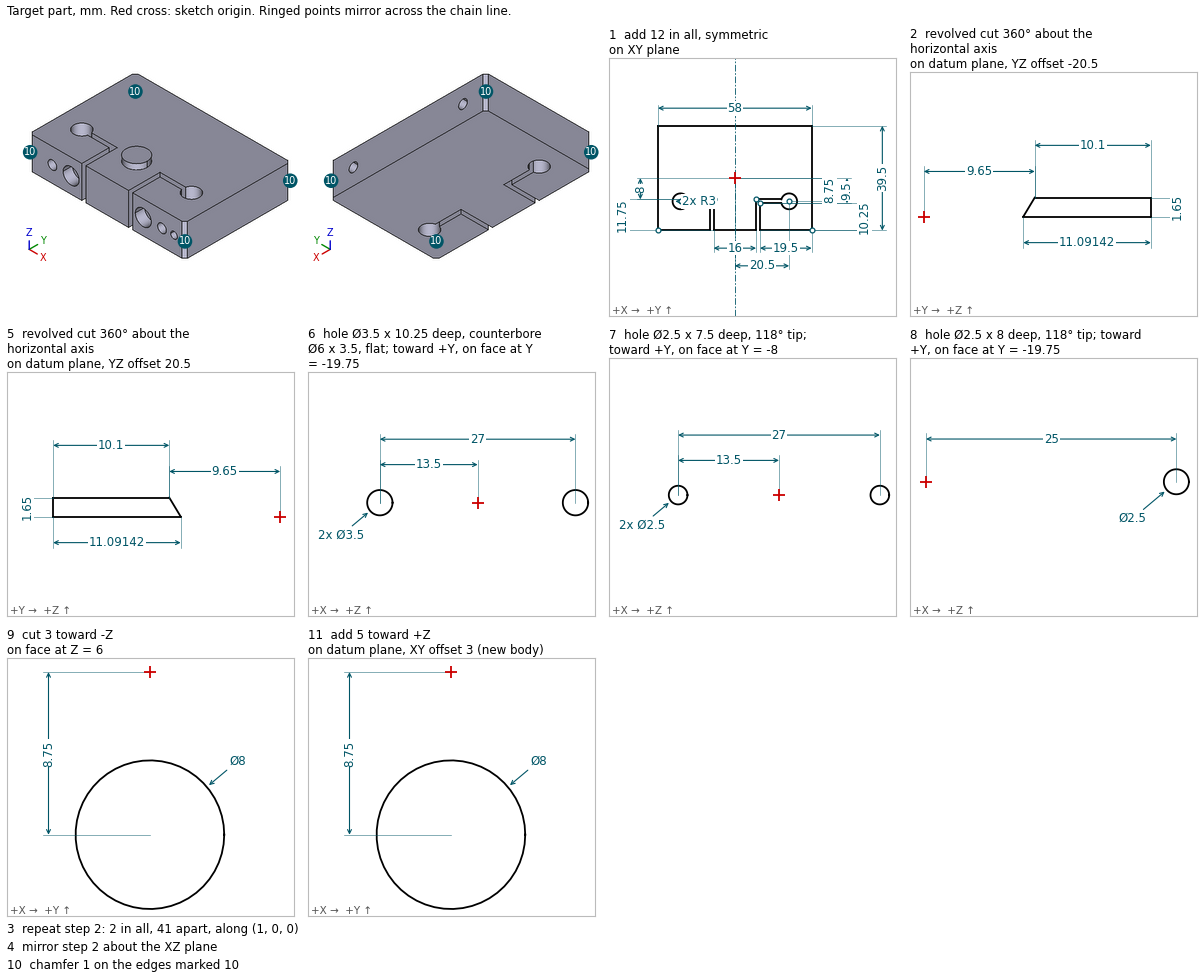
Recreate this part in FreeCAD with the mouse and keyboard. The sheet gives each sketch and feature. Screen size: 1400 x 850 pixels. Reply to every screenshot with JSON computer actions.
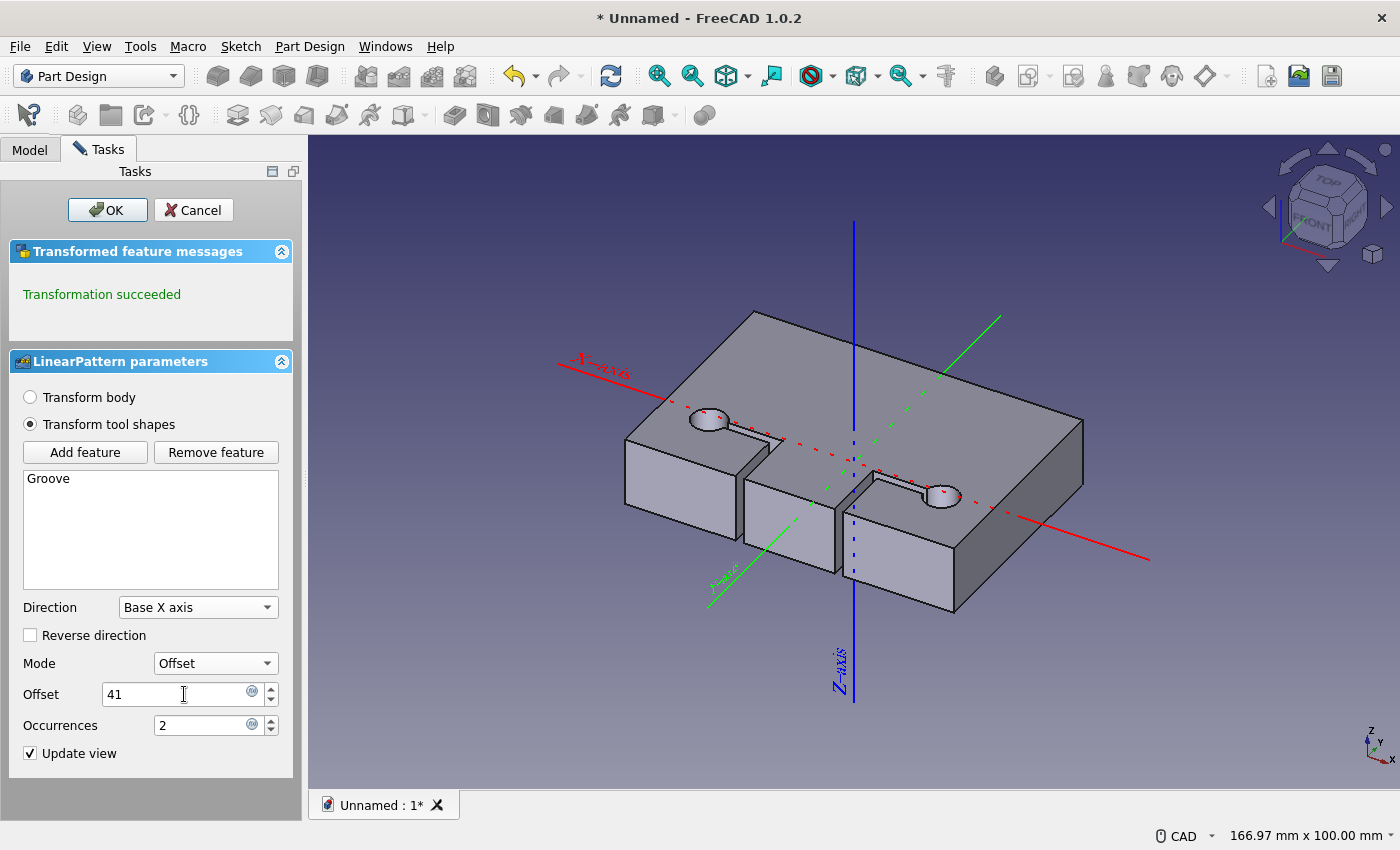
{"action": "triple_click", "coordinate": [210, 726]}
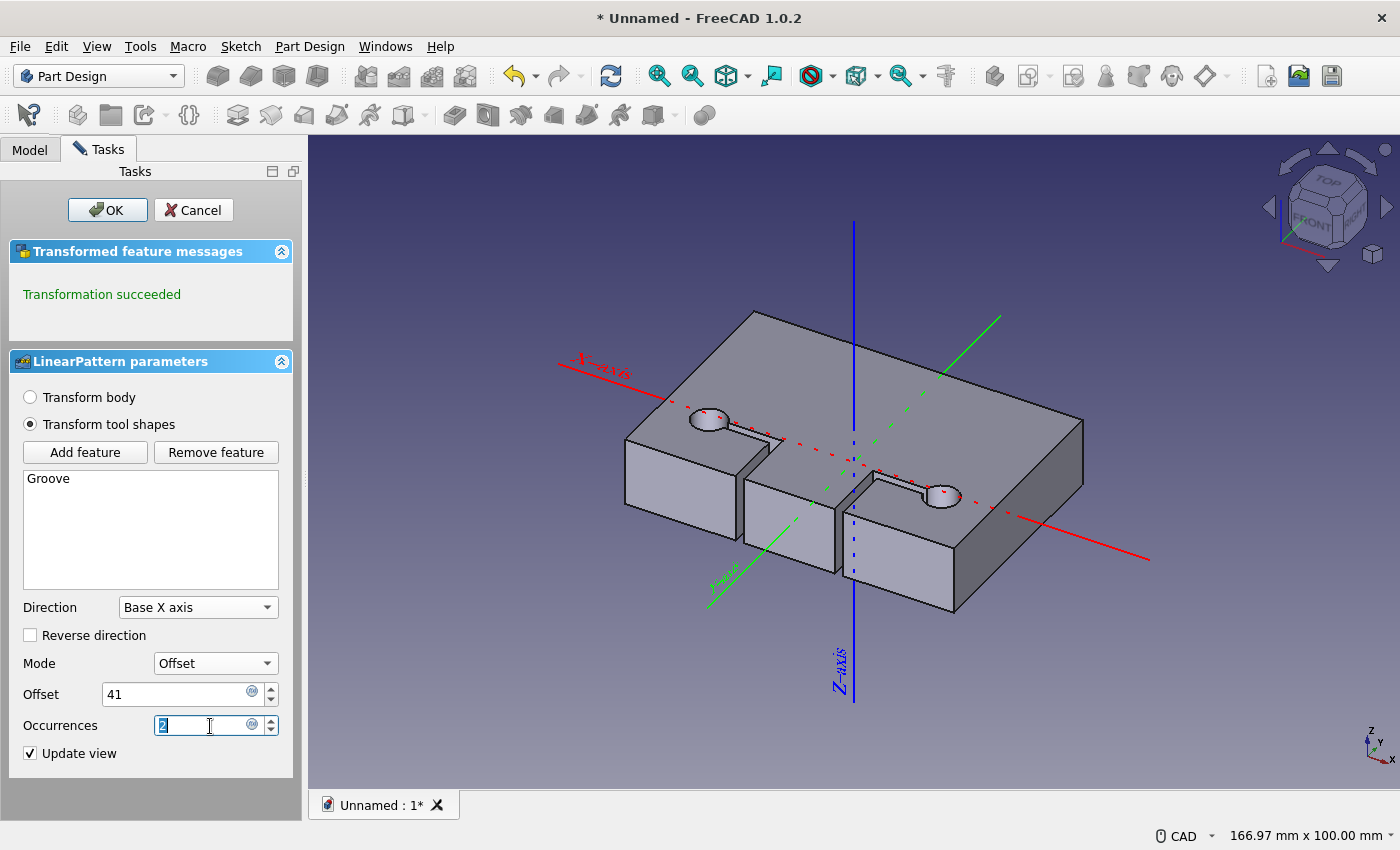
{"action": "type", "text": "2"}
{"action": "key", "text": "Tab"}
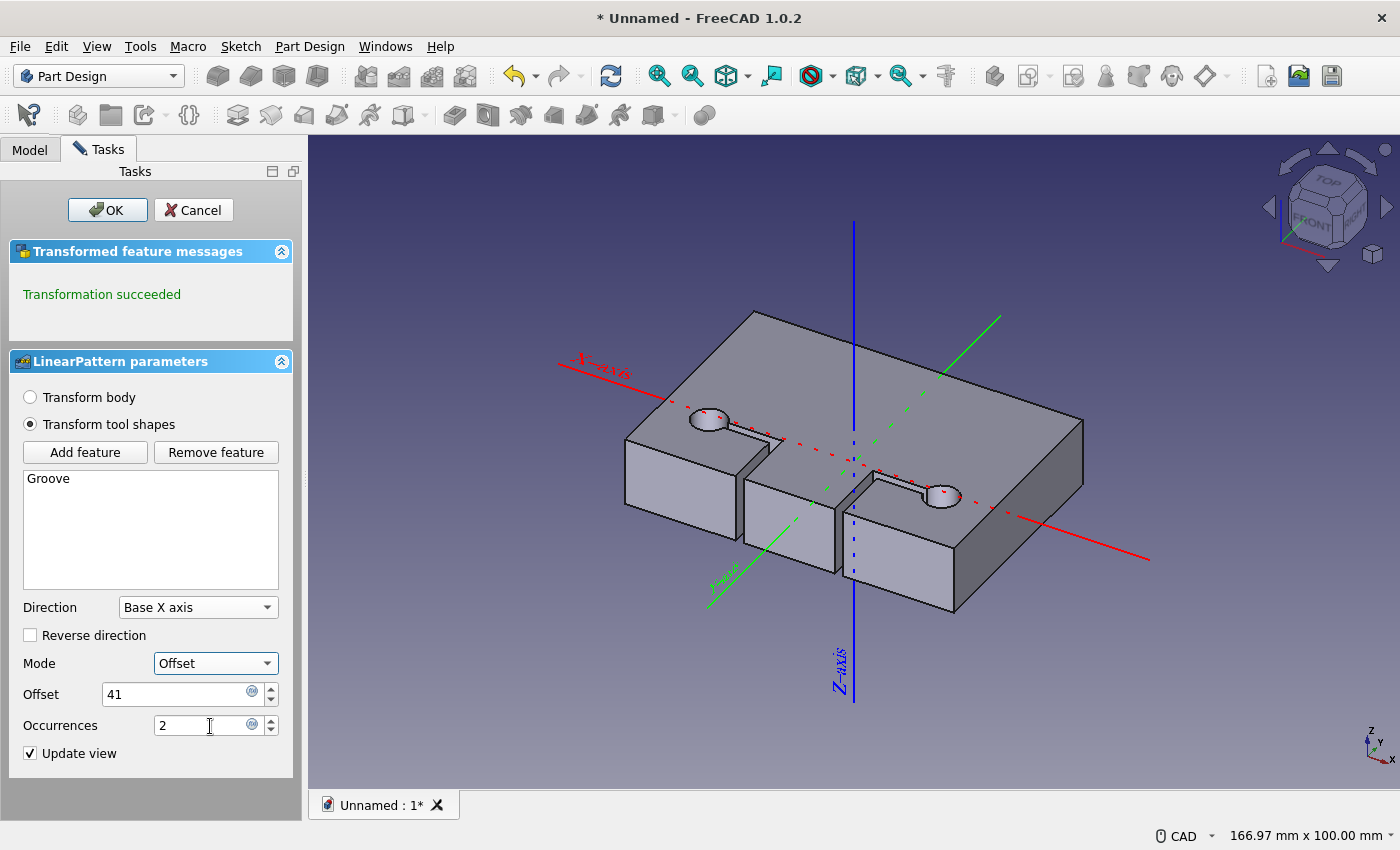
{"action": "left_click", "coordinate": [108, 210]}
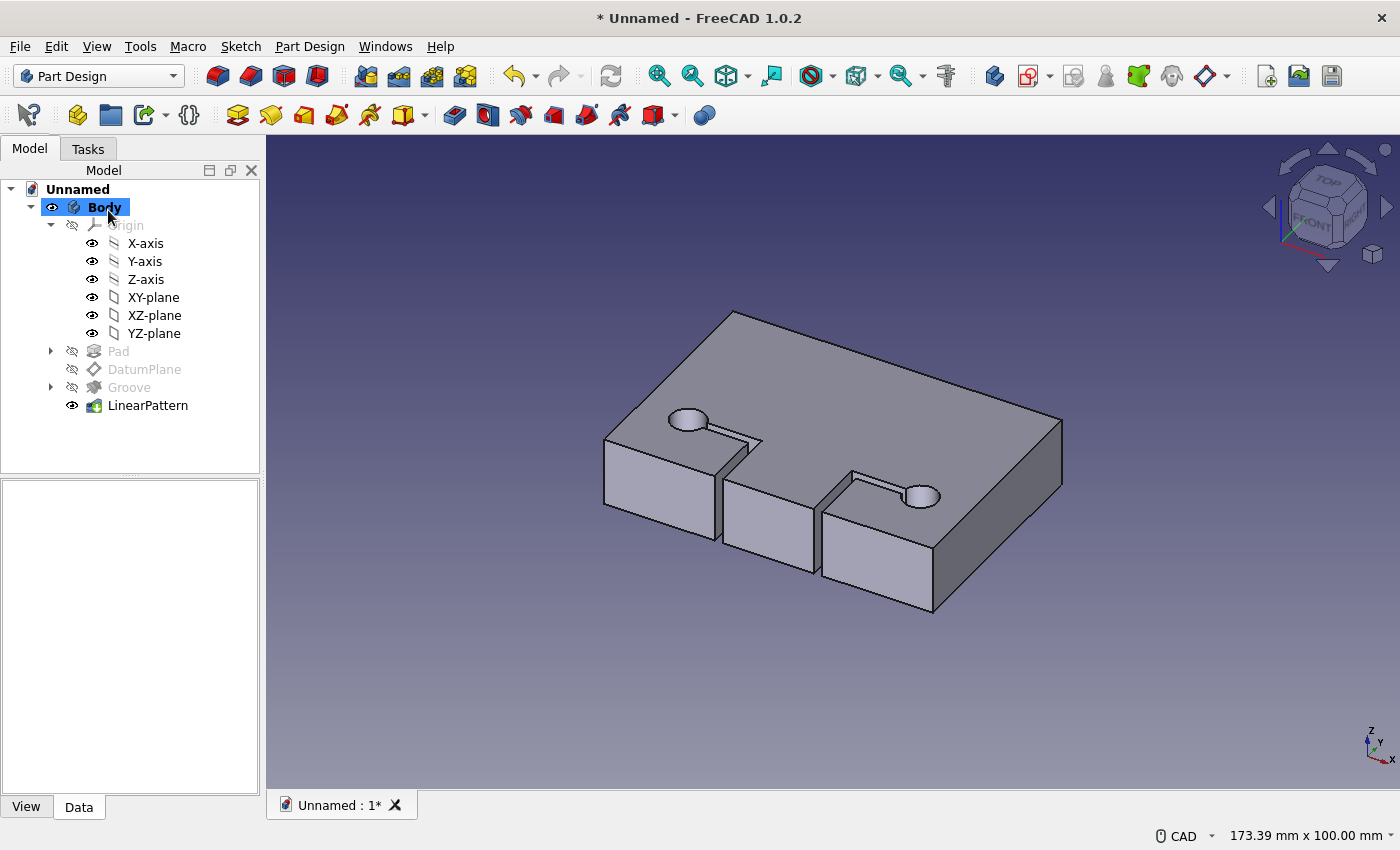
{"action": "left_click", "coordinate": [117, 387]}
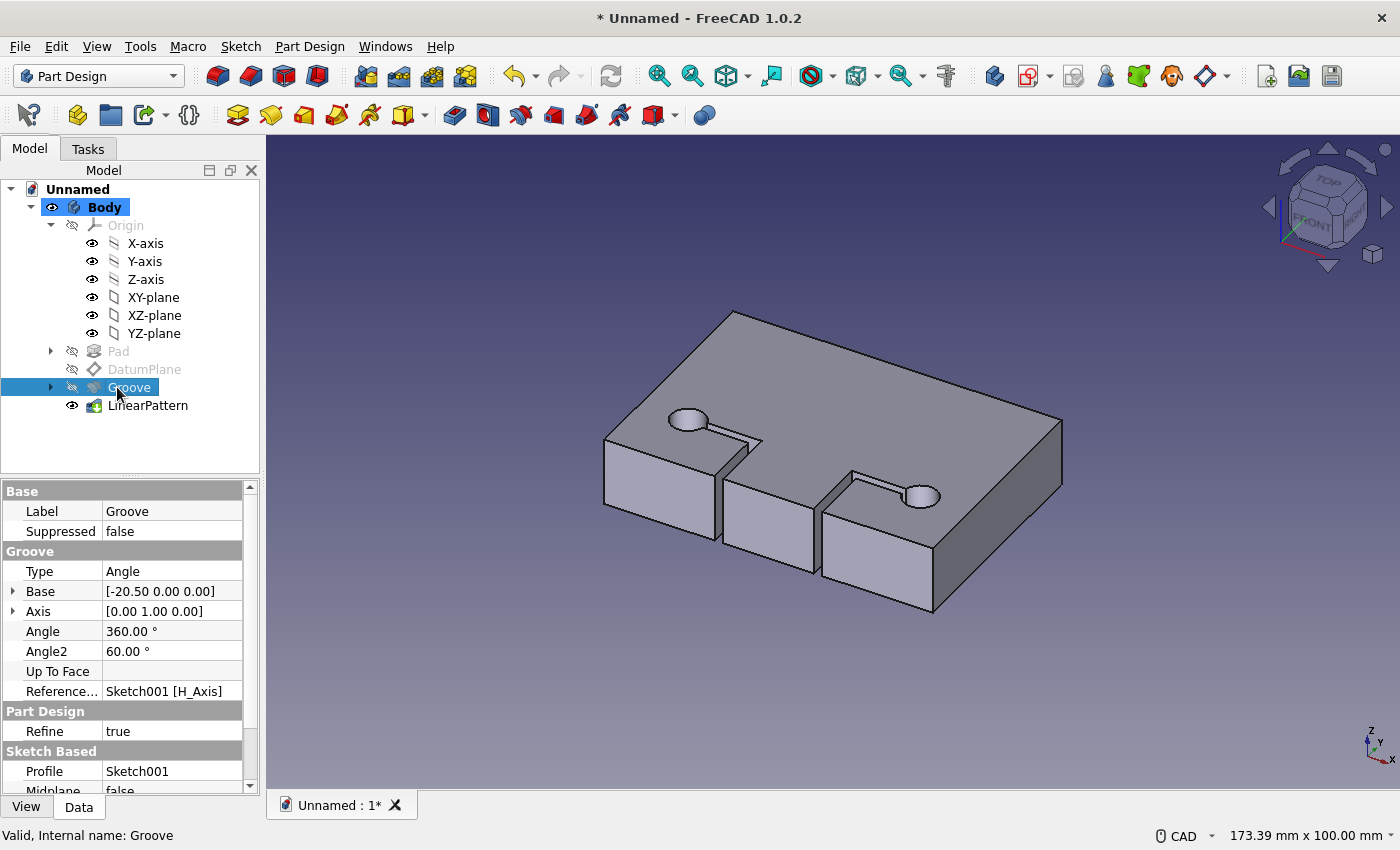
{"action": "left_click", "coordinate": [366, 76]}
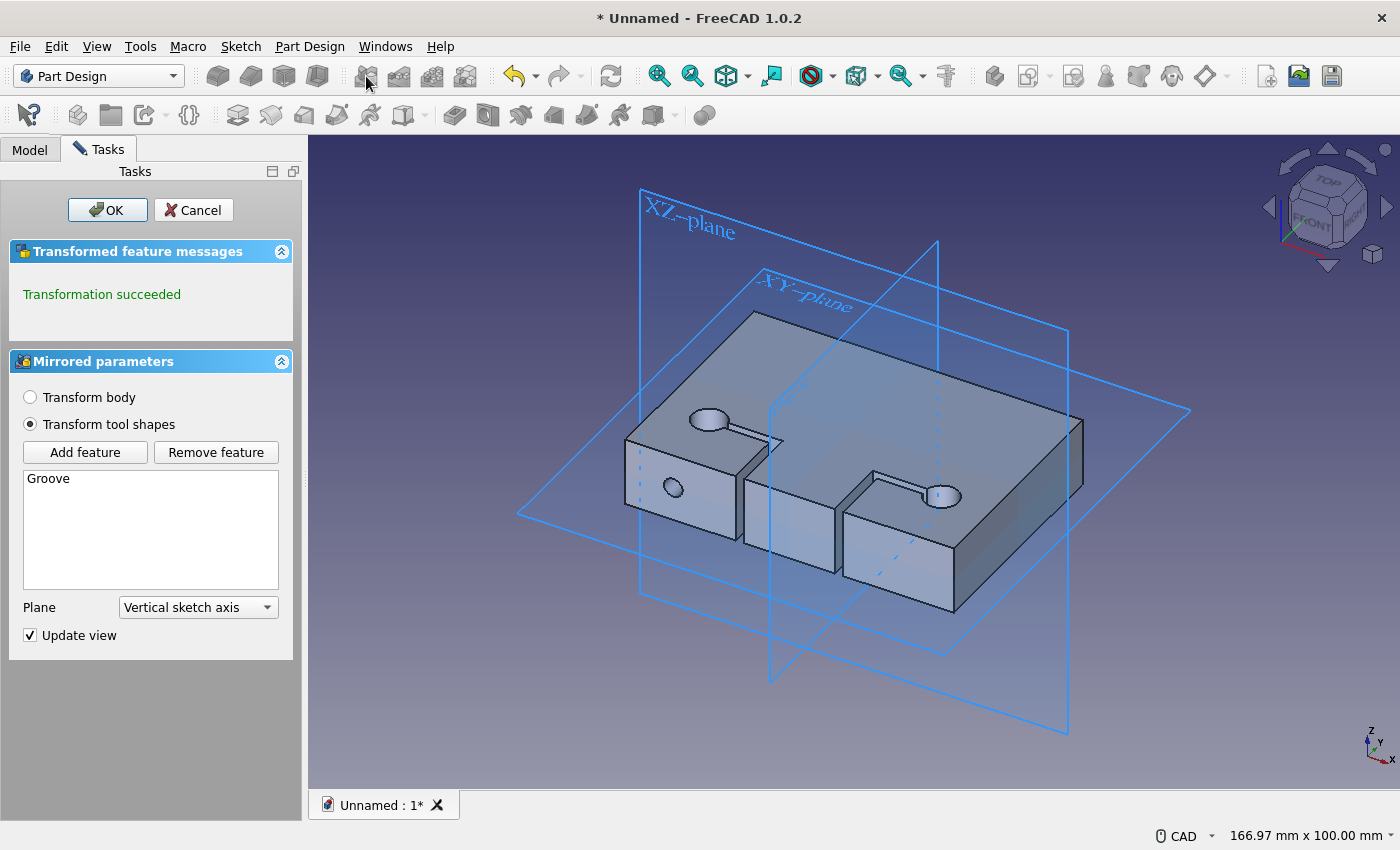
{"action": "left_click", "coordinate": [199, 608]}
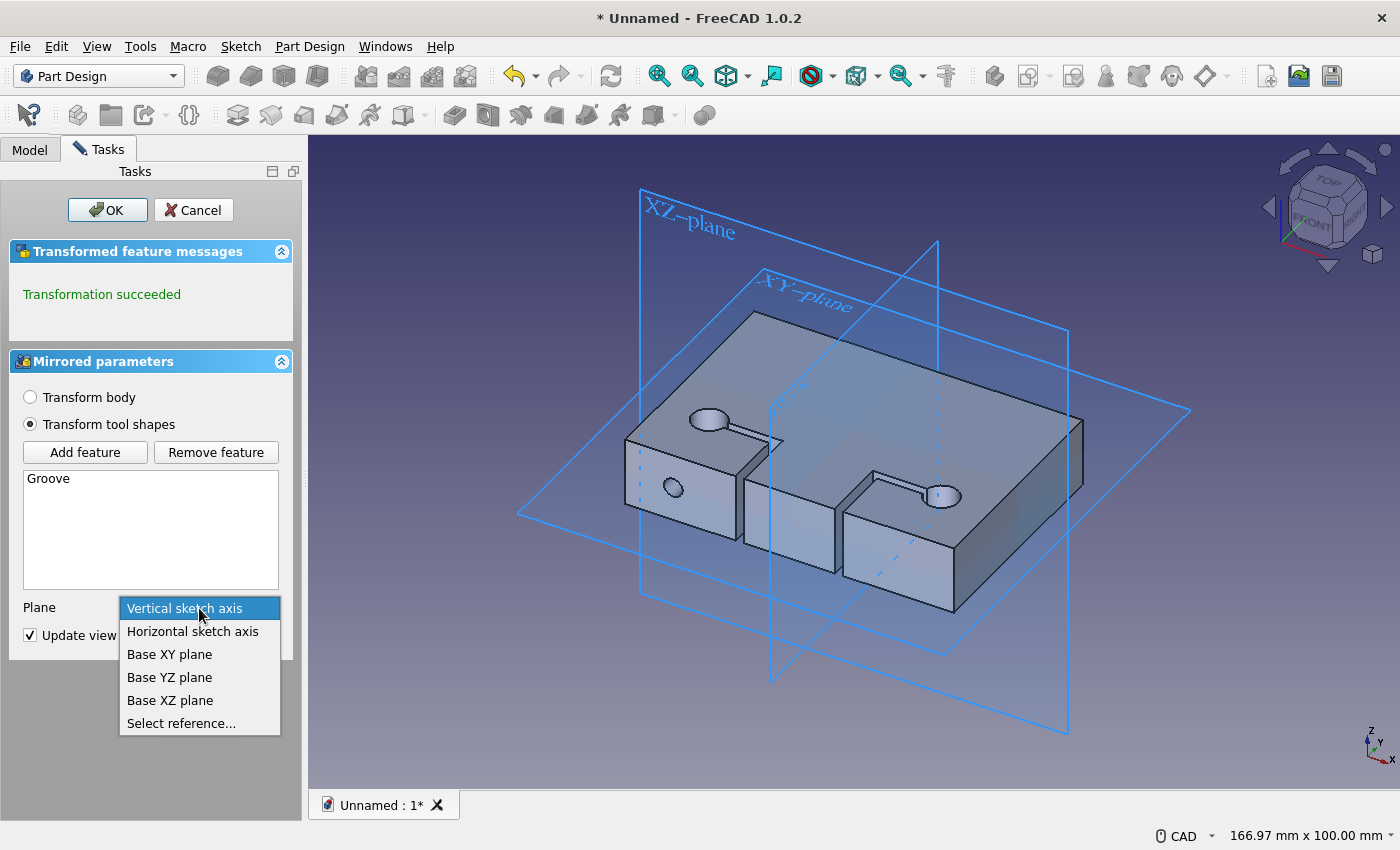
{"action": "left_click", "coordinate": [198, 700]}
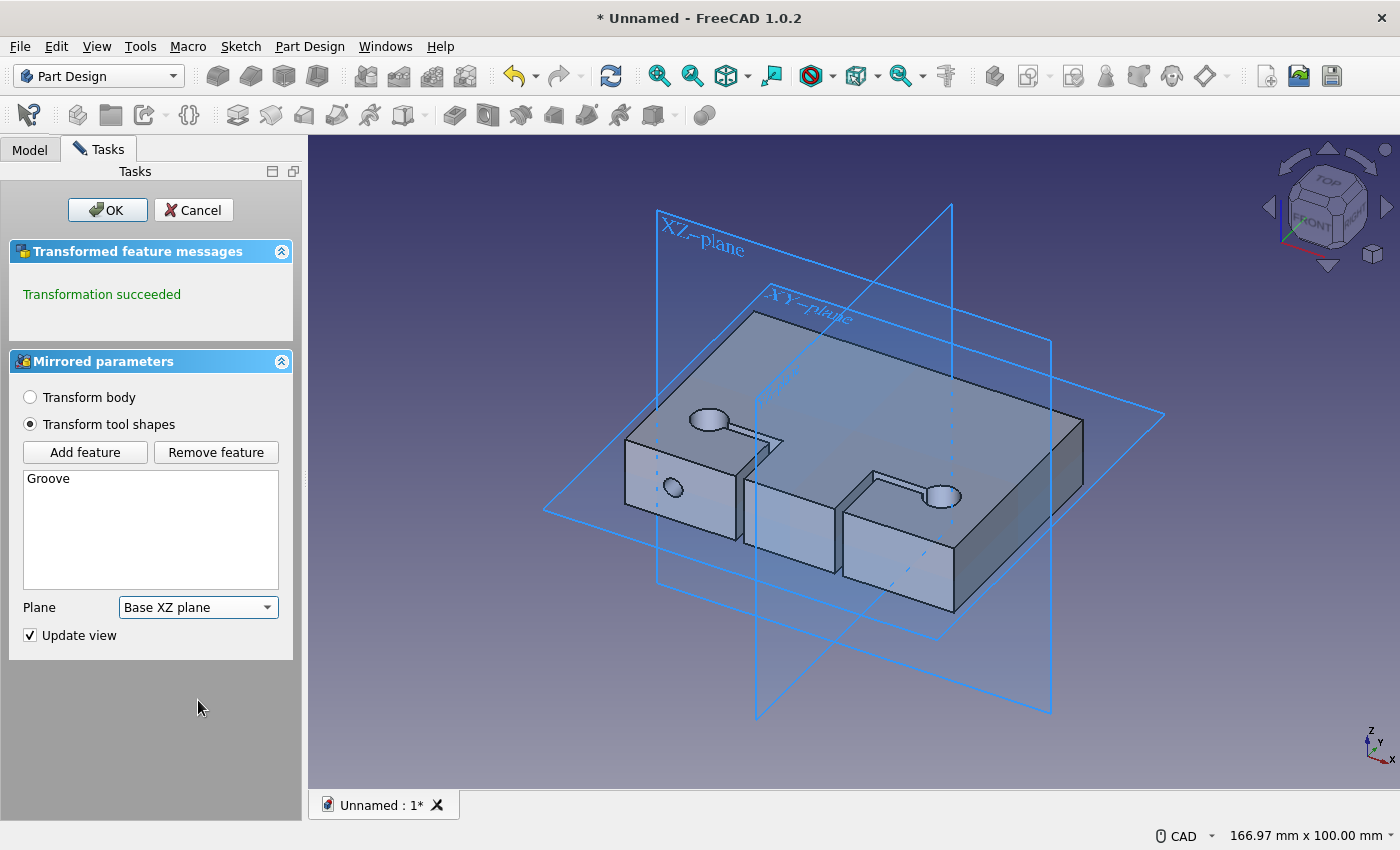
{"action": "left_click", "coordinate": [108, 210]}